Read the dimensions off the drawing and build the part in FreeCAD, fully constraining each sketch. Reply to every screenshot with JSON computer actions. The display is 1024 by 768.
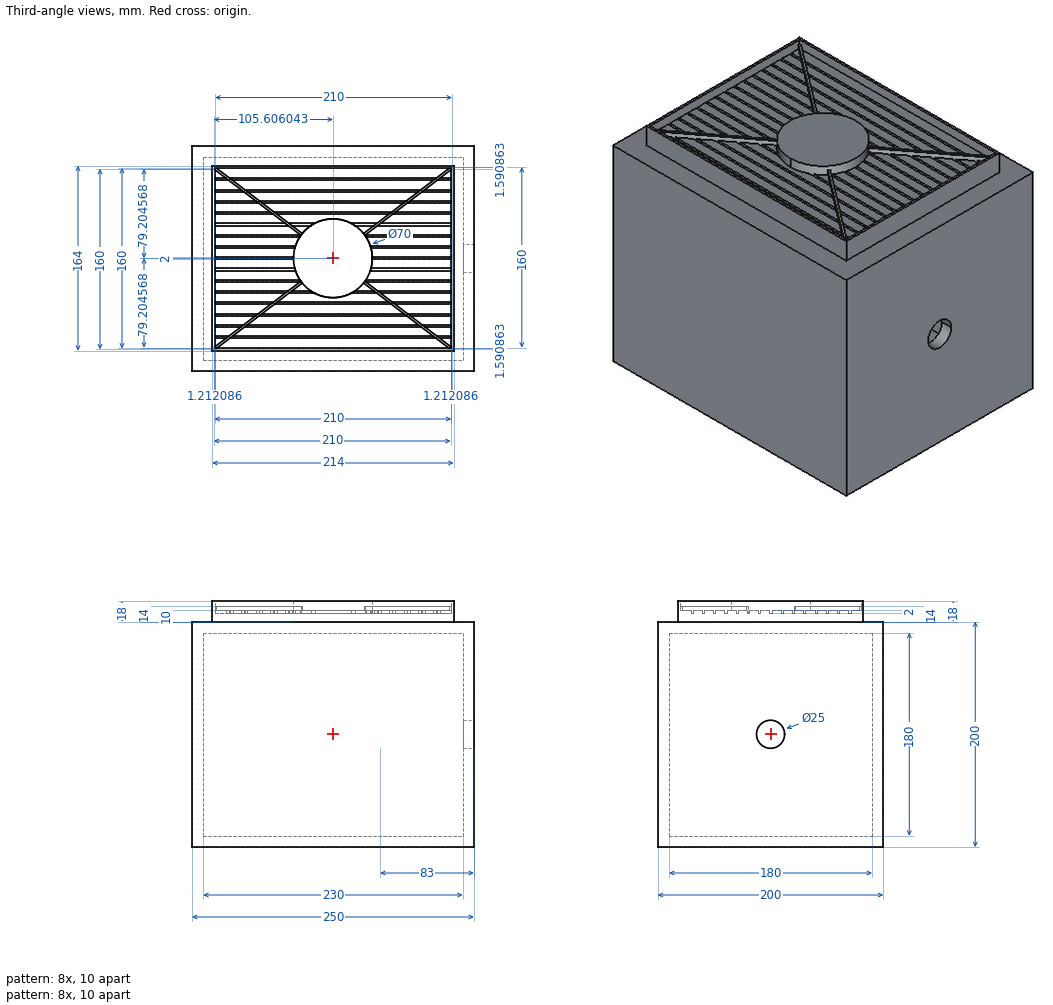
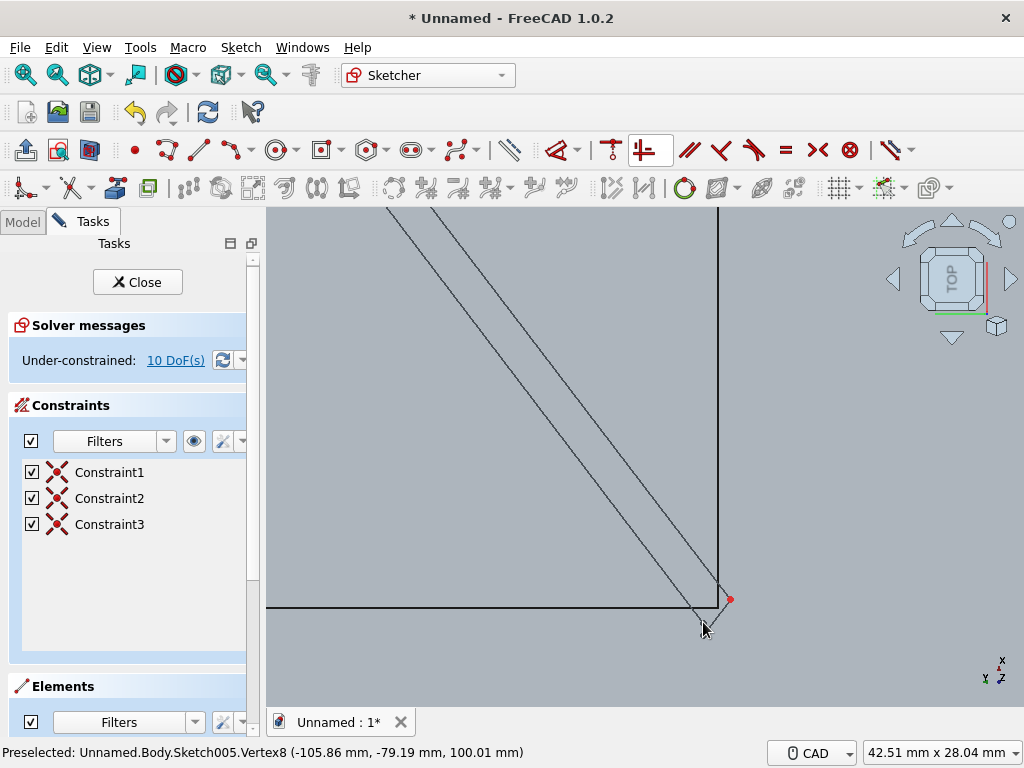
{"action": "left_click", "coordinate": [556, 150]}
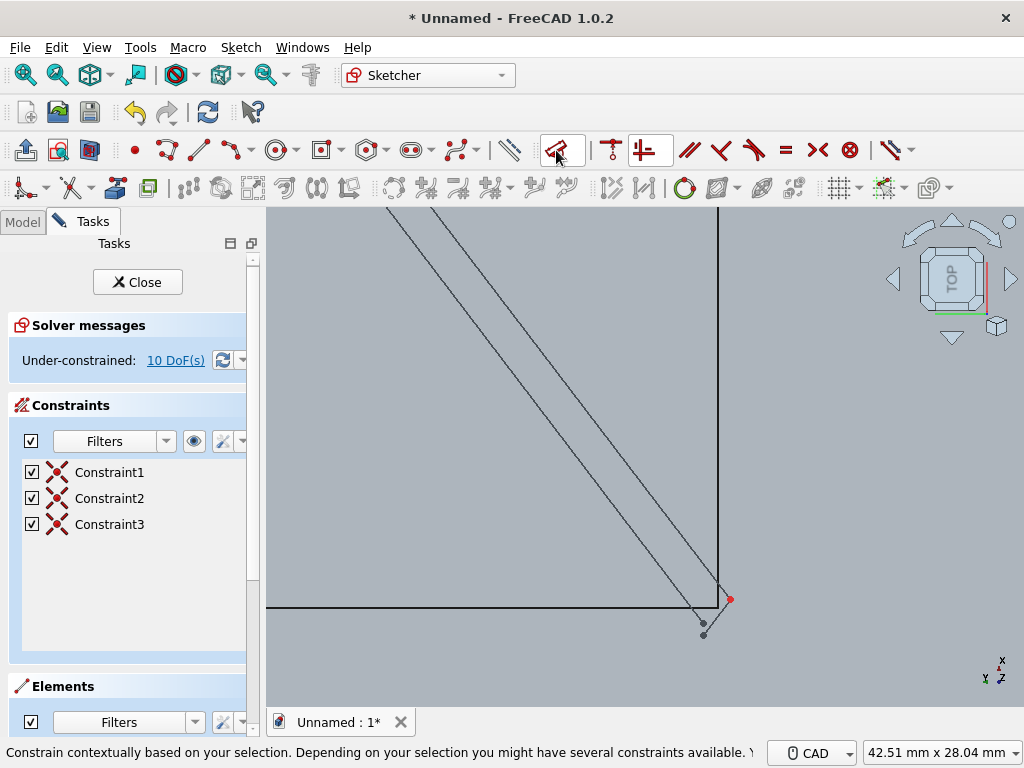
{"action": "scroll", "coordinate": [705, 629], "scroll_direction": "down", "scroll_amount": 12}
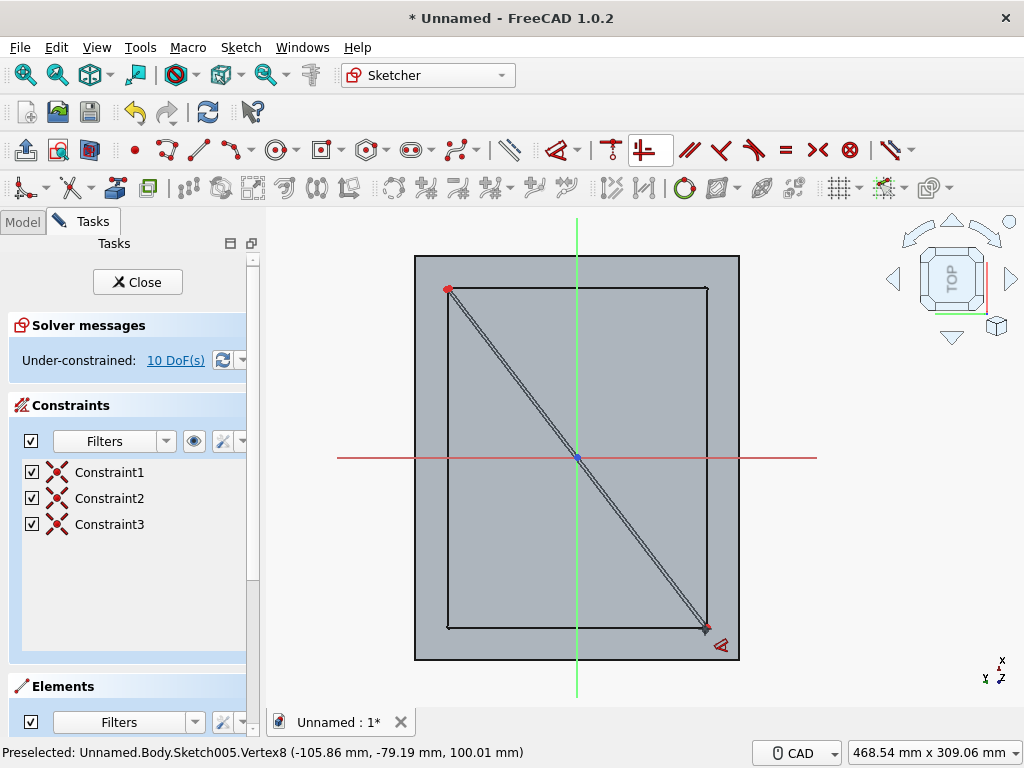
{"action": "scroll", "coordinate": [630, 525], "scroll_direction": "up", "scroll_amount": 8}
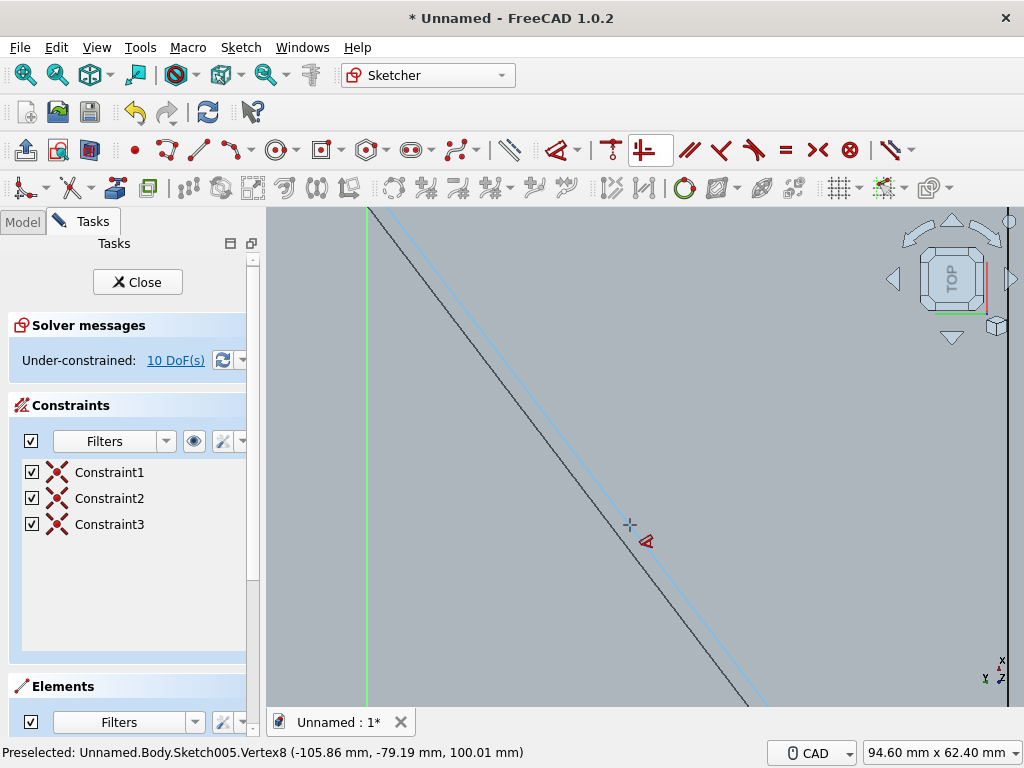
{"action": "left_click", "coordinate": [629, 525]}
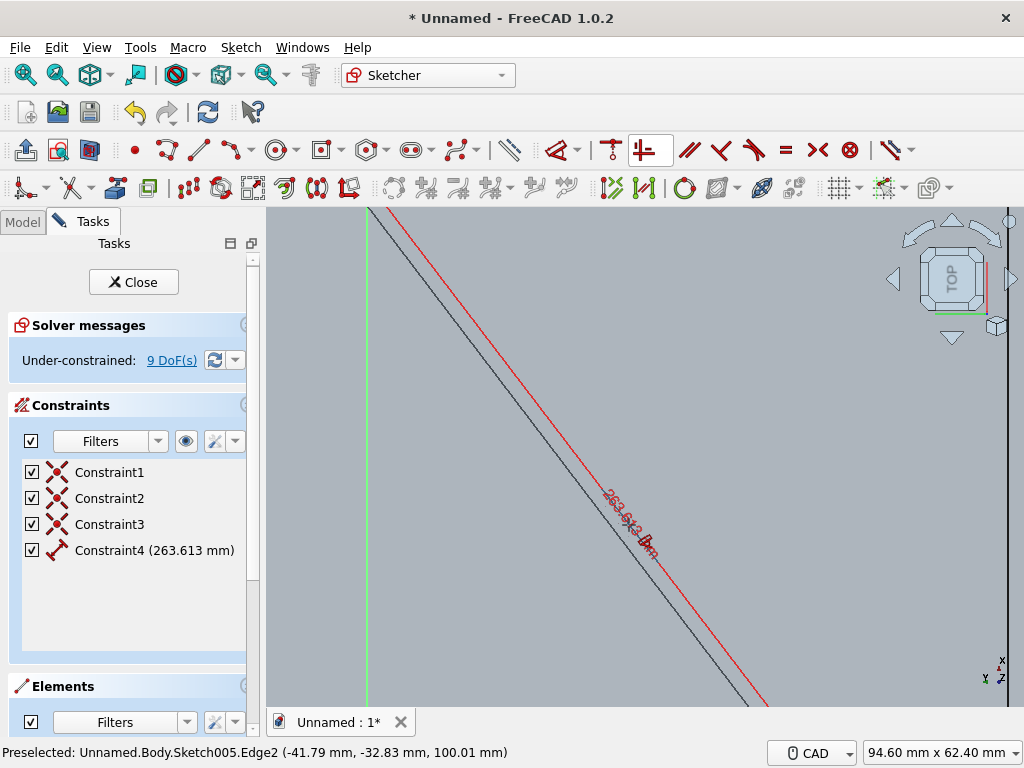
{"action": "key", "text": "Escape"}
{"action": "key", "text": "Escape"}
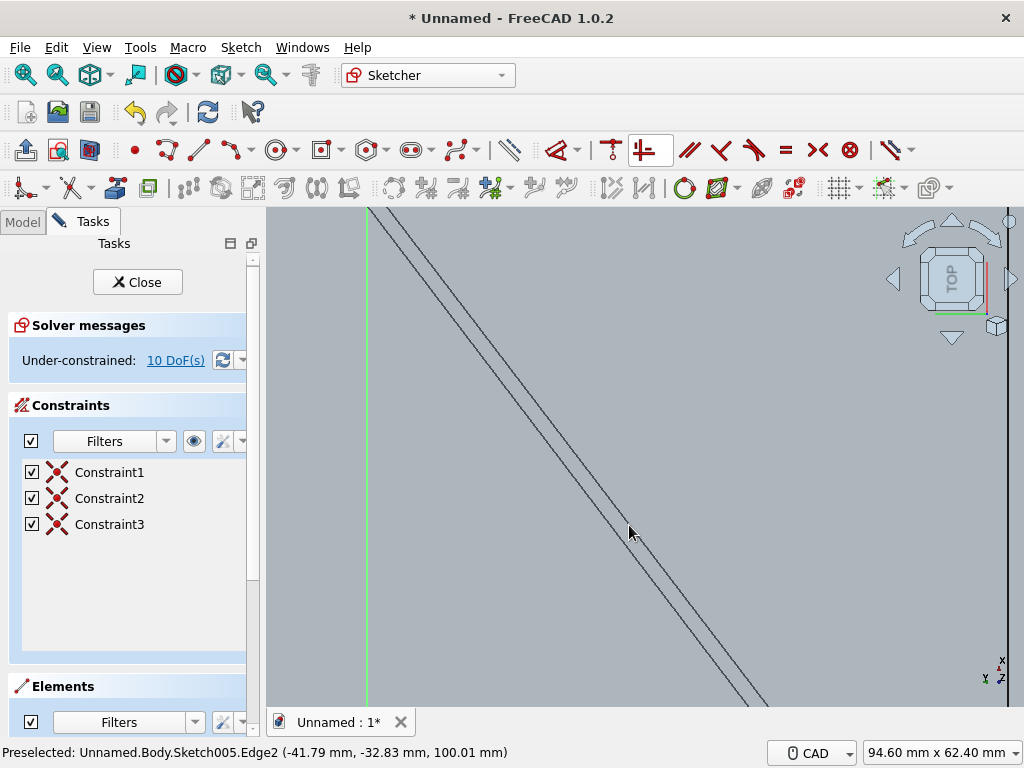
{"action": "left_click", "coordinate": [629, 525]}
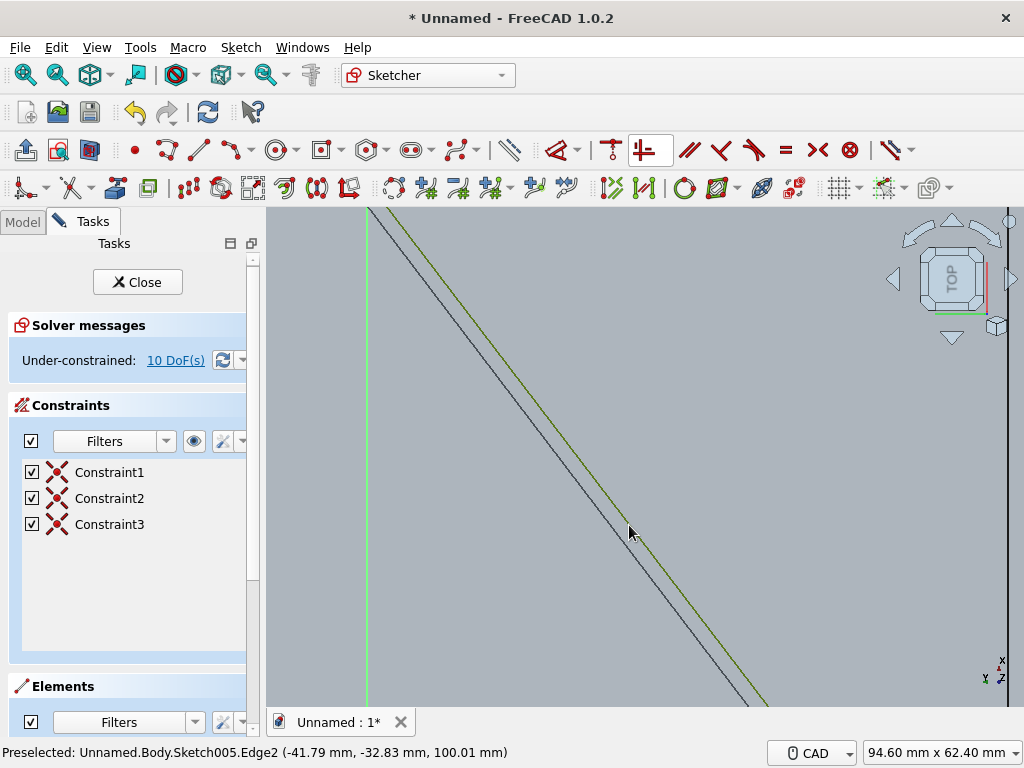
{"action": "left_click", "coordinate": [580, 150]}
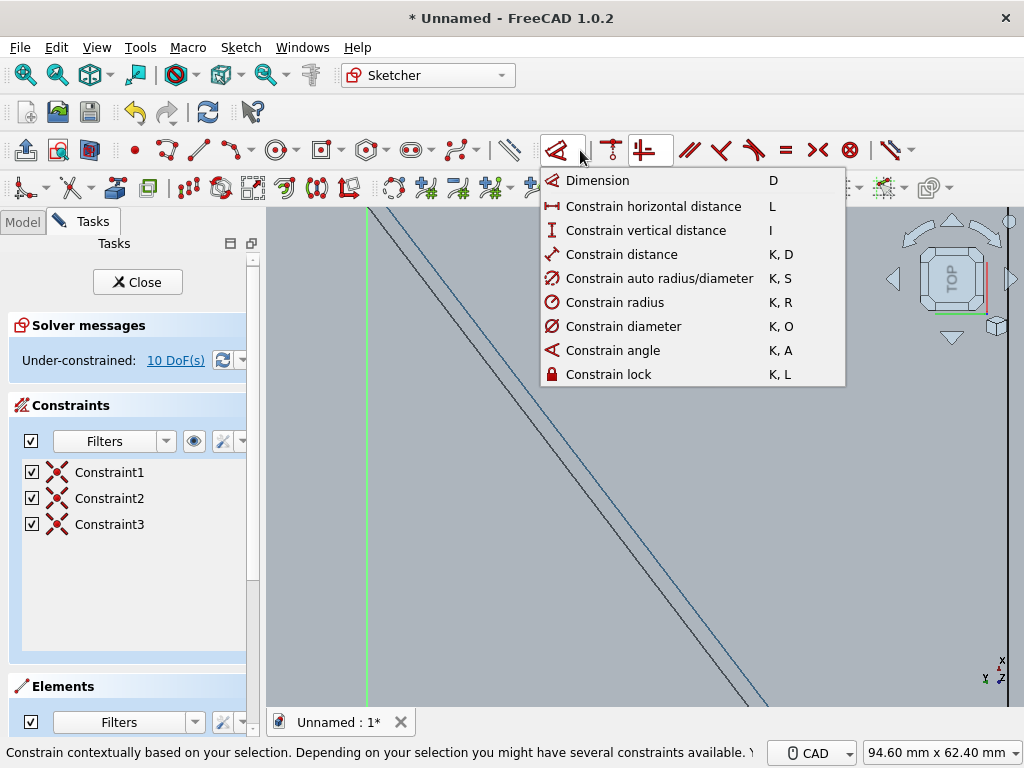
{"action": "left_click", "coordinate": [693, 206]}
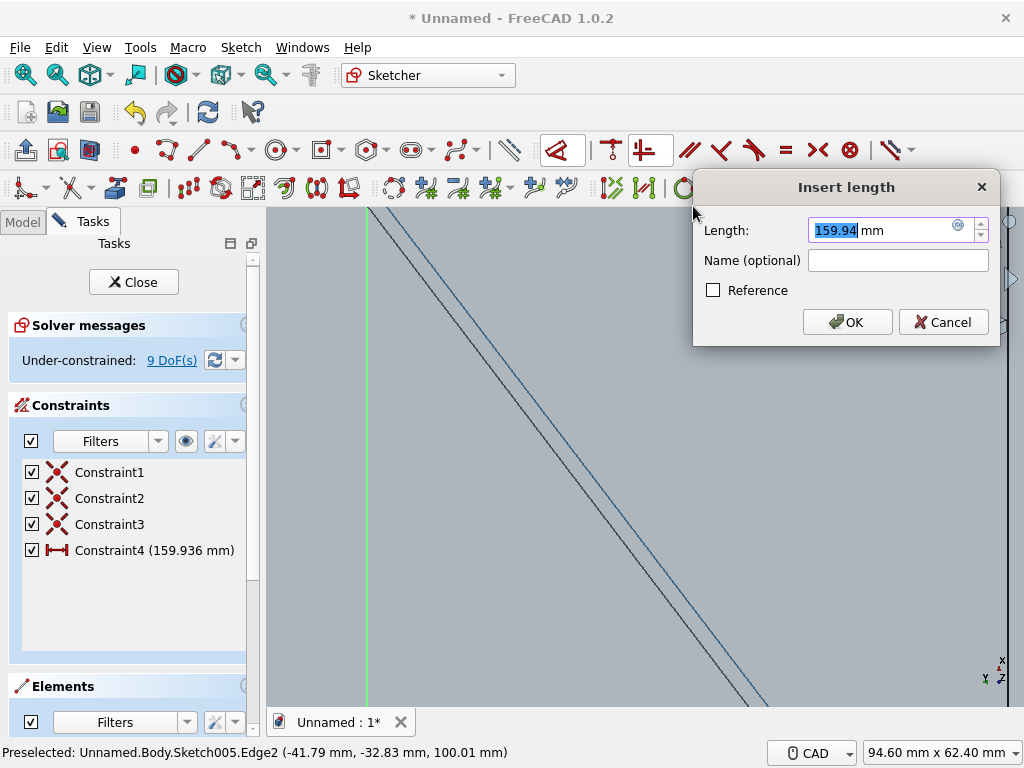
{"action": "type", "text": "160"}
{"action": "key", "text": "Return"}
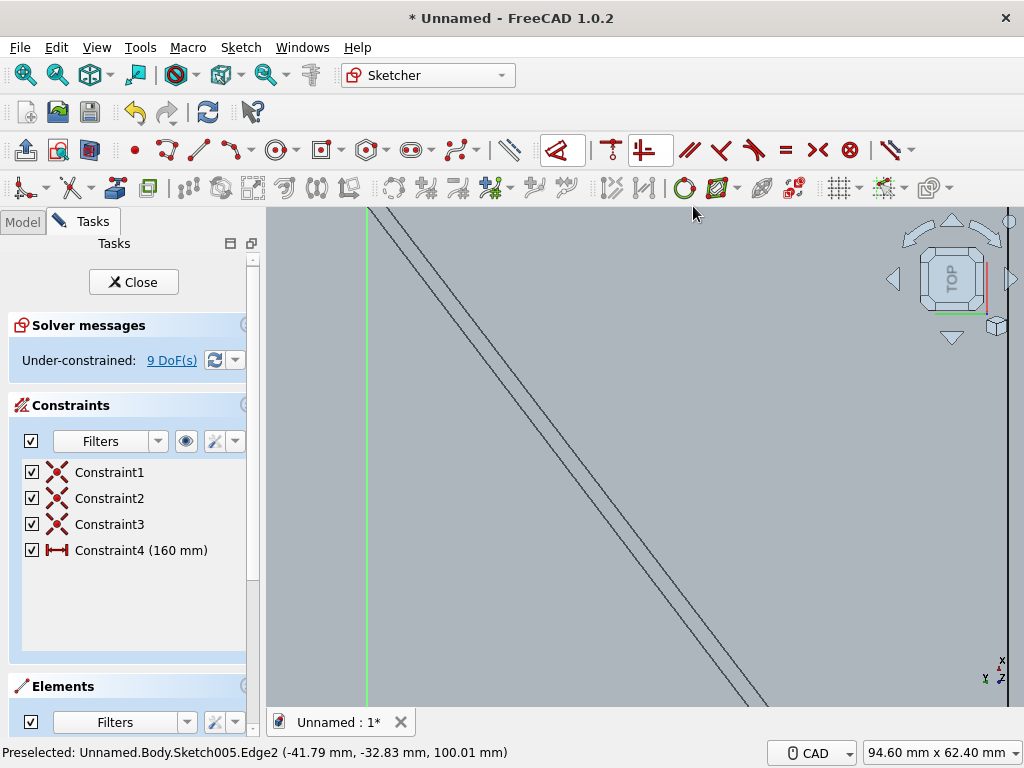
{"action": "left_click", "coordinate": [629, 525]}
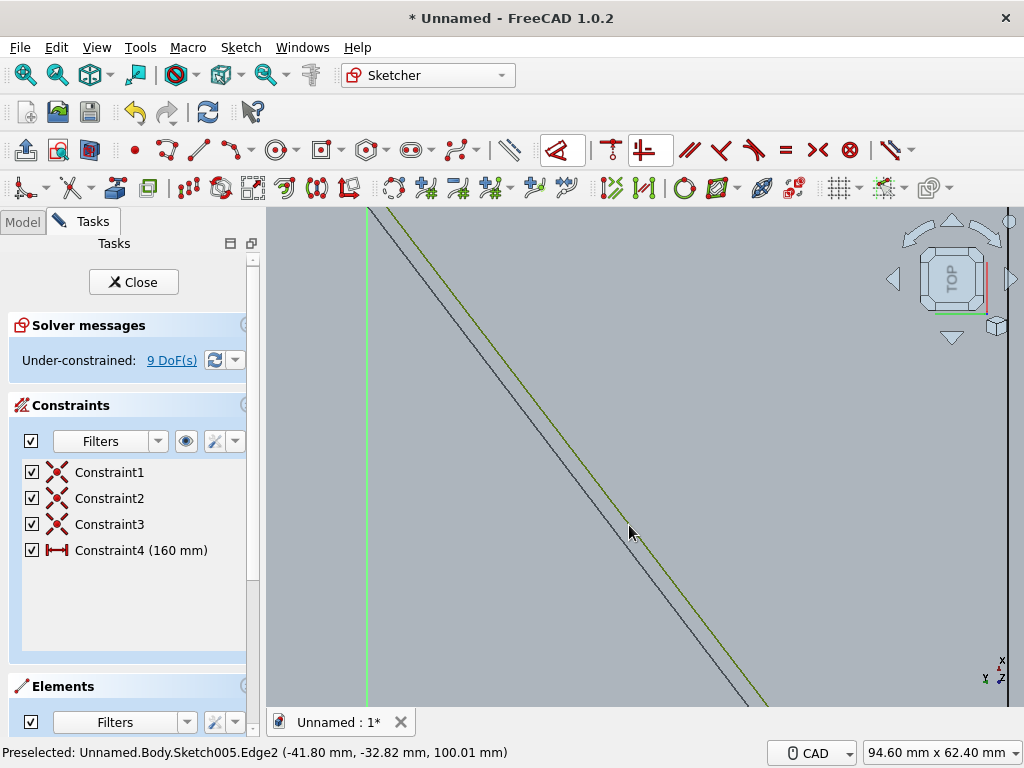
{"action": "left_click", "coordinate": [580, 150]}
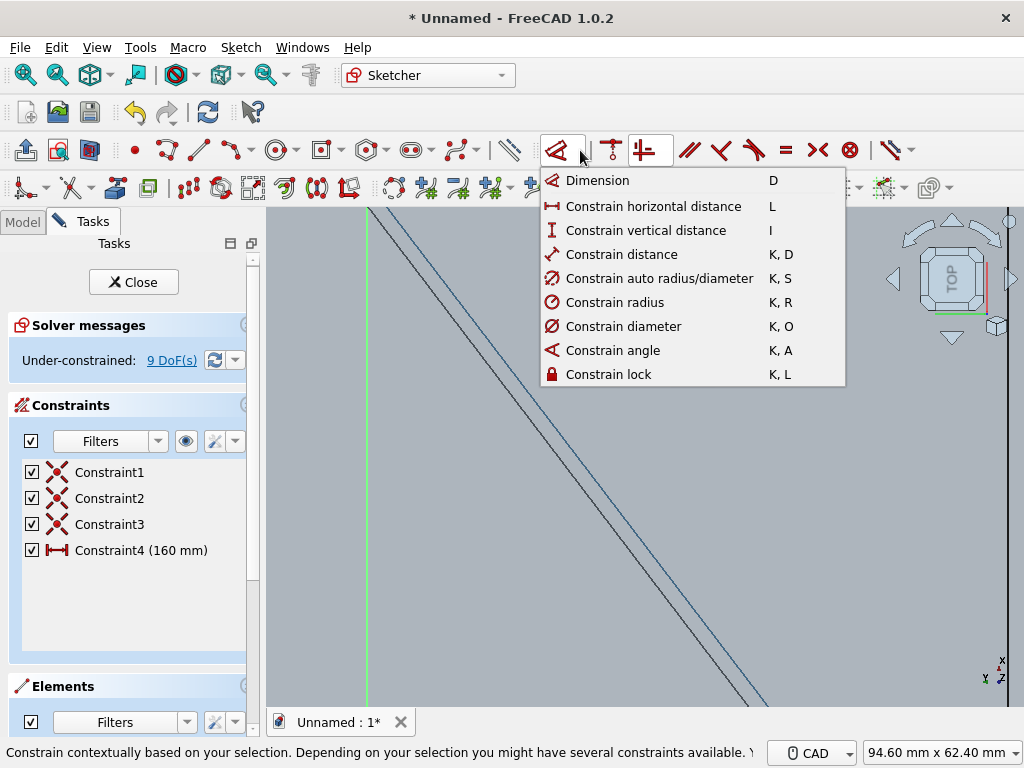
{"action": "left_click", "coordinate": [693, 230]}